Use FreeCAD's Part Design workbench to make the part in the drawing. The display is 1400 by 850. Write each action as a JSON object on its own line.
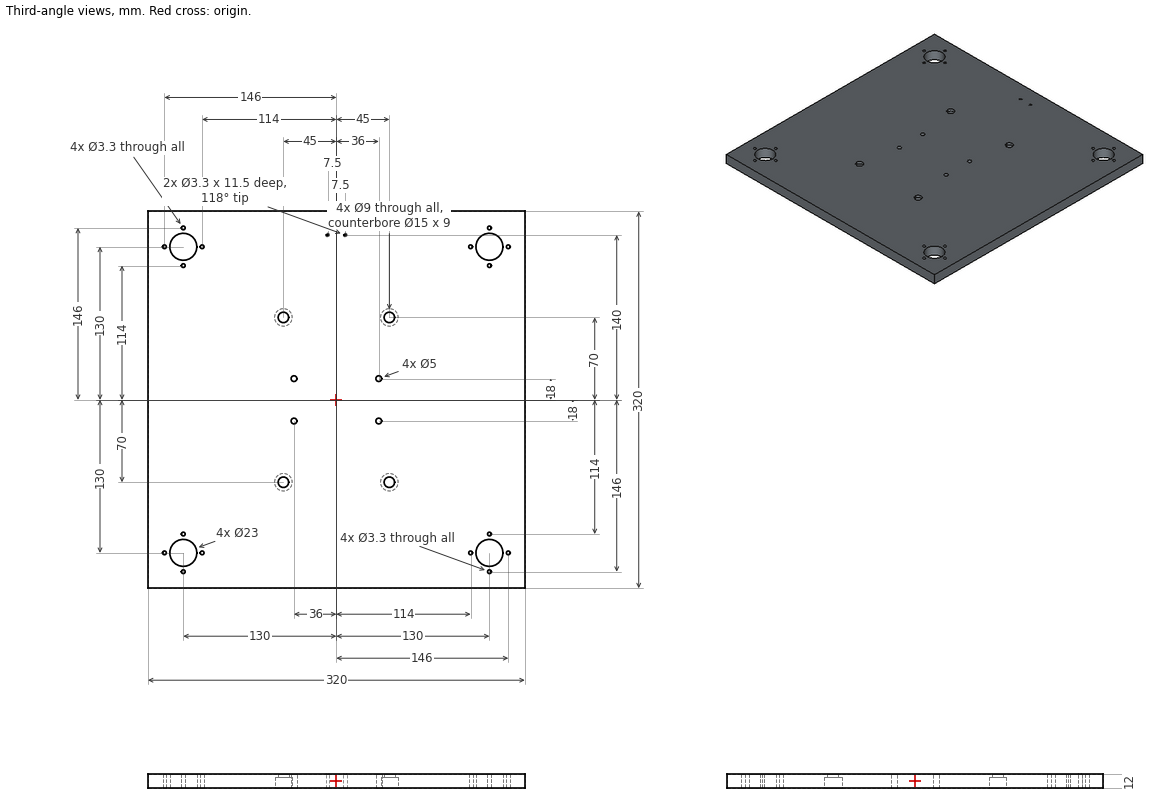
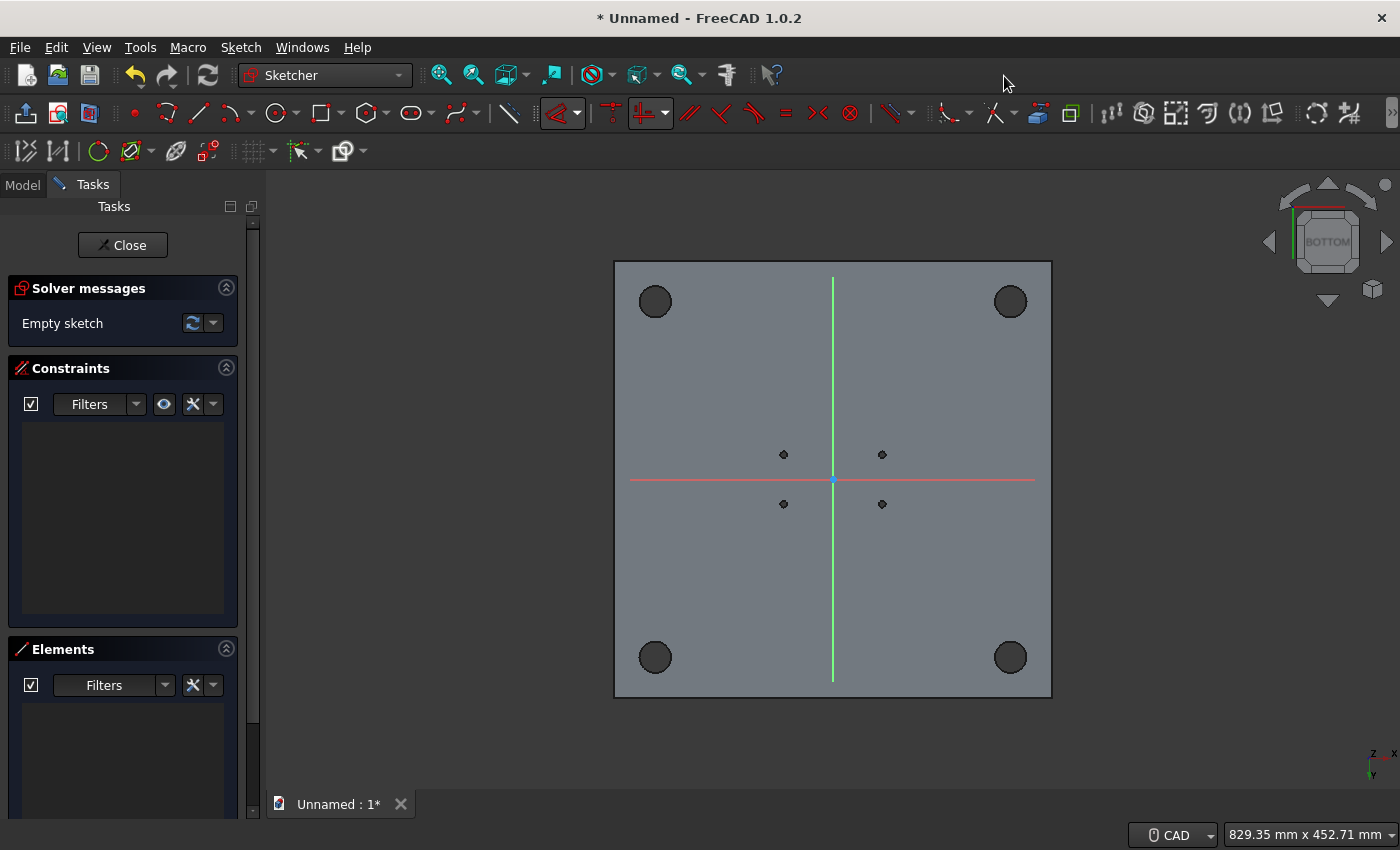
{"action": "scroll", "coordinate": [916, 480], "scroll_direction": "up", "scroll_amount": 3}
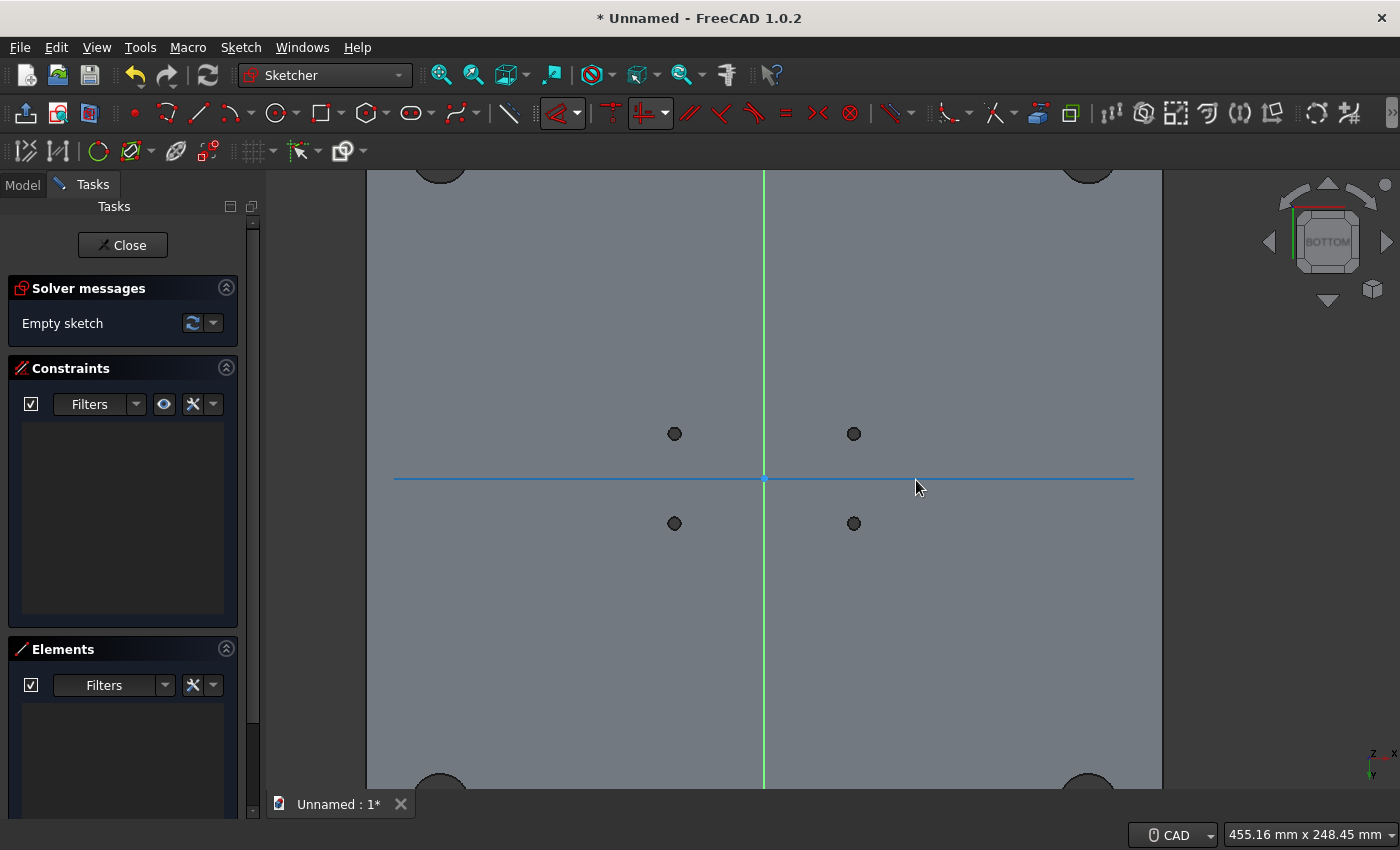
{"action": "left_click", "coordinate": [276, 114]}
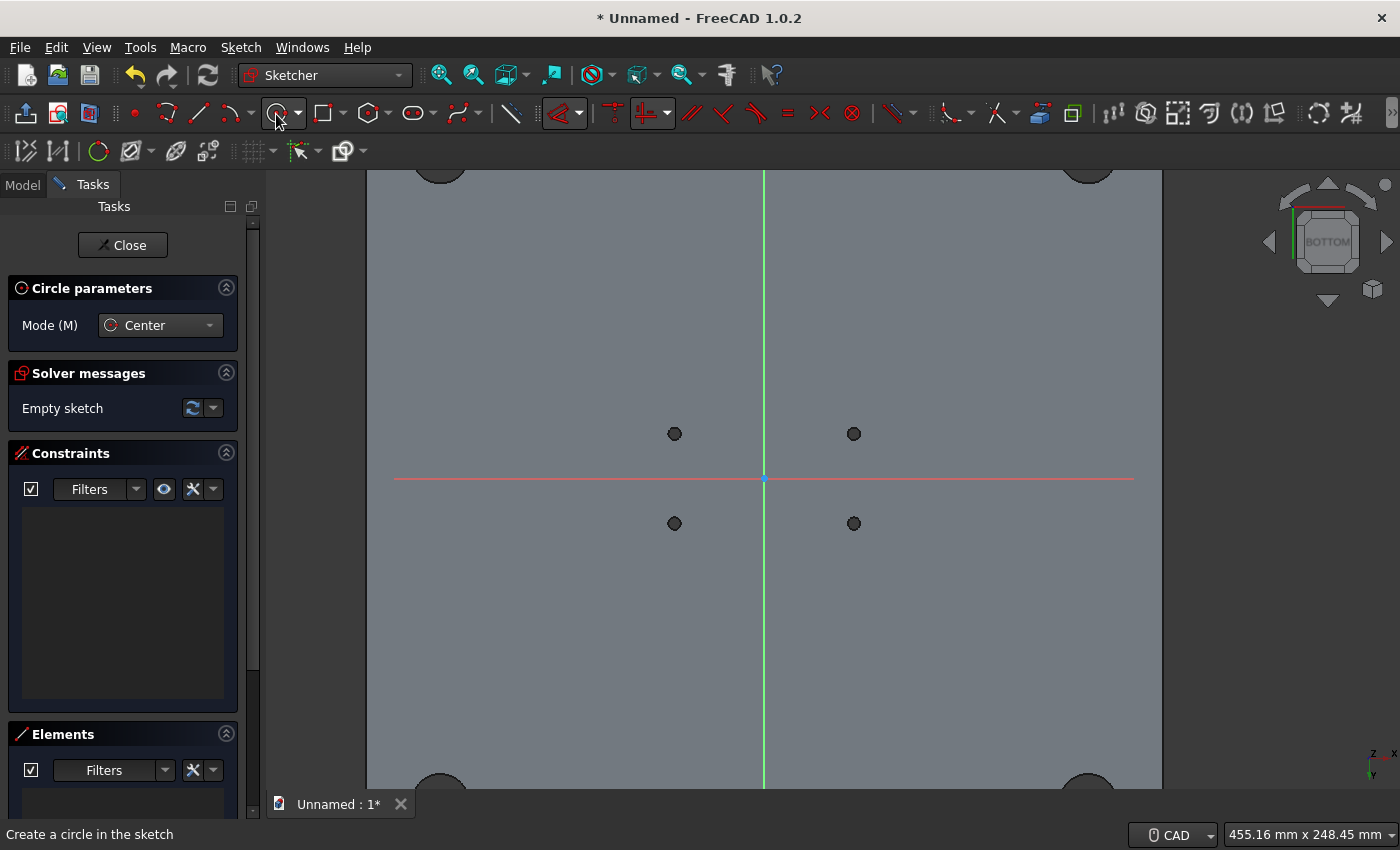
{"action": "scroll", "coordinate": [876, 653], "scroll_direction": "up", "scroll_amount": 4}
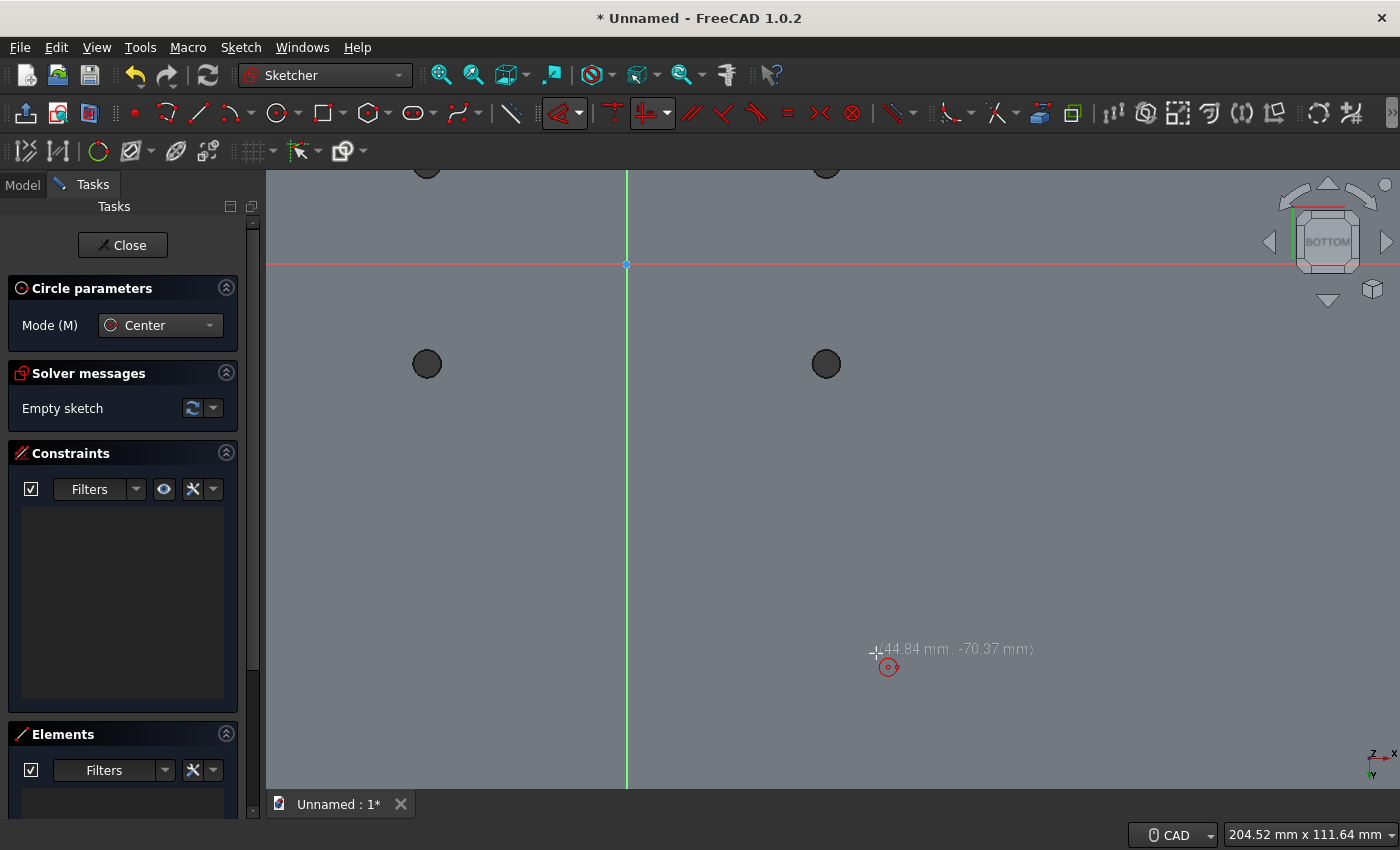
{"action": "left_click", "coordinate": [876, 652]}
{"action": "mouse_move", "coordinate": [894, 635]}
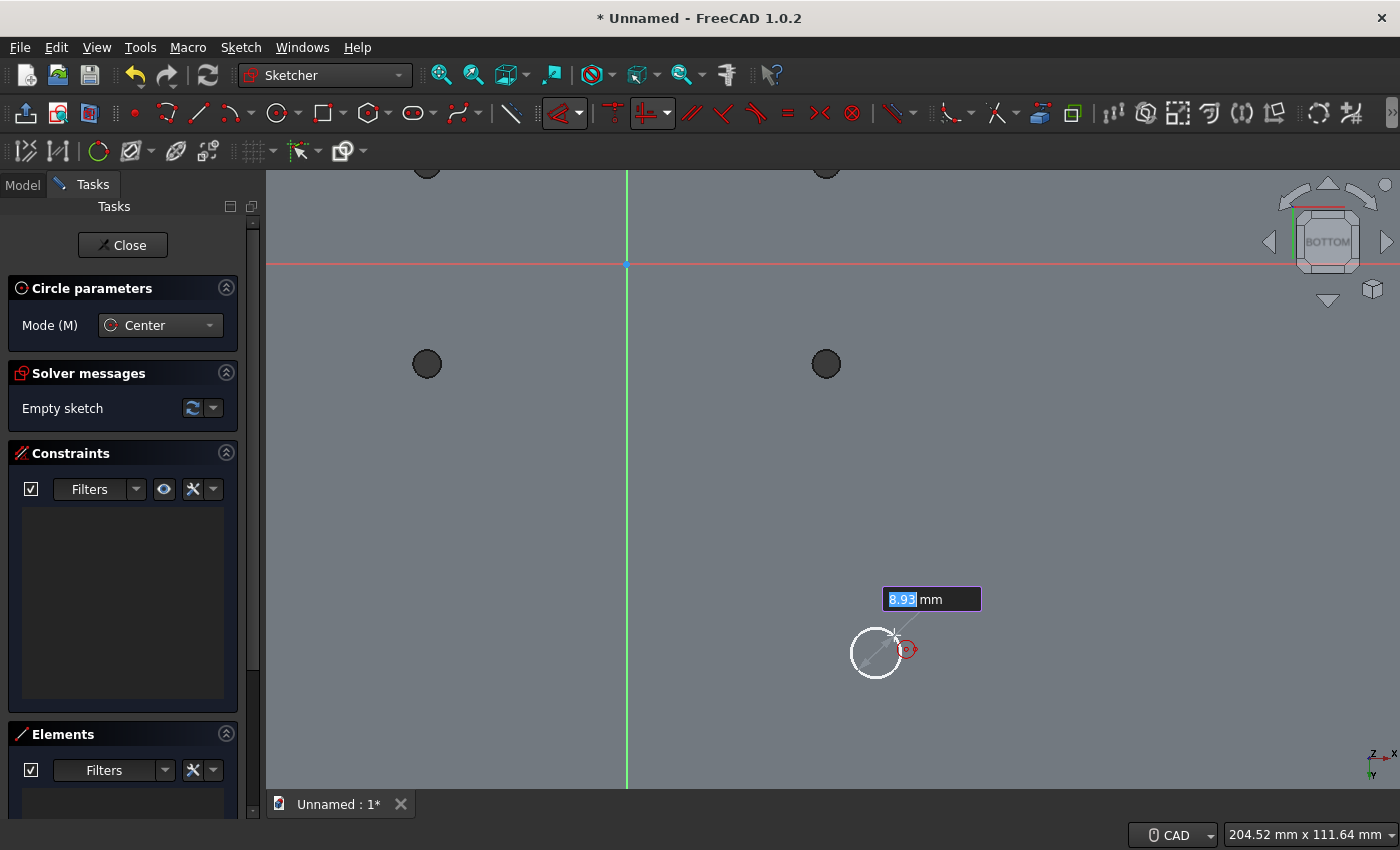
{"action": "type", "text": "9"}
{"action": "key", "text": "Return"}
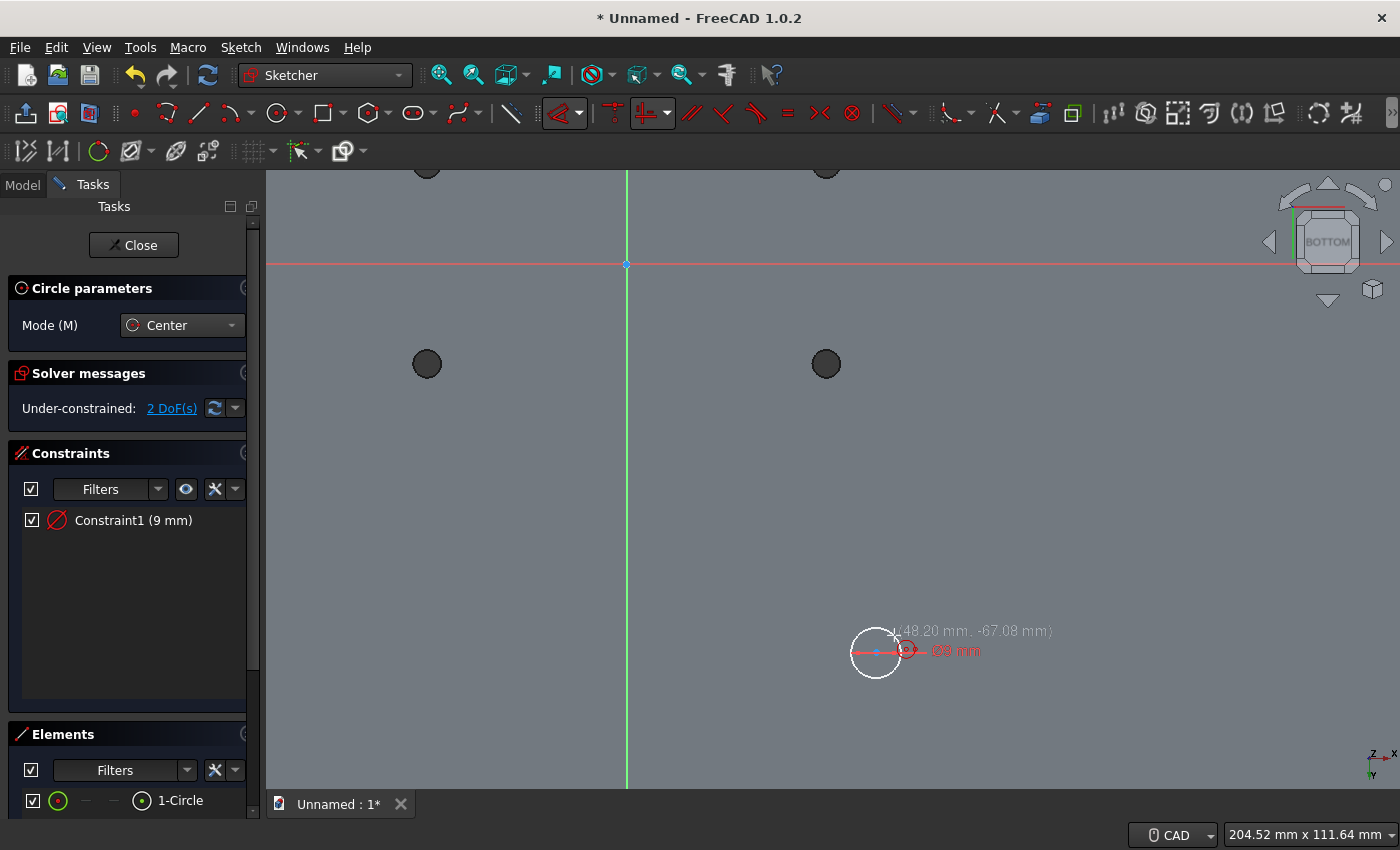
{"action": "left_click", "coordinate": [377, 652]}
{"action": "mouse_move", "coordinate": [395, 635]}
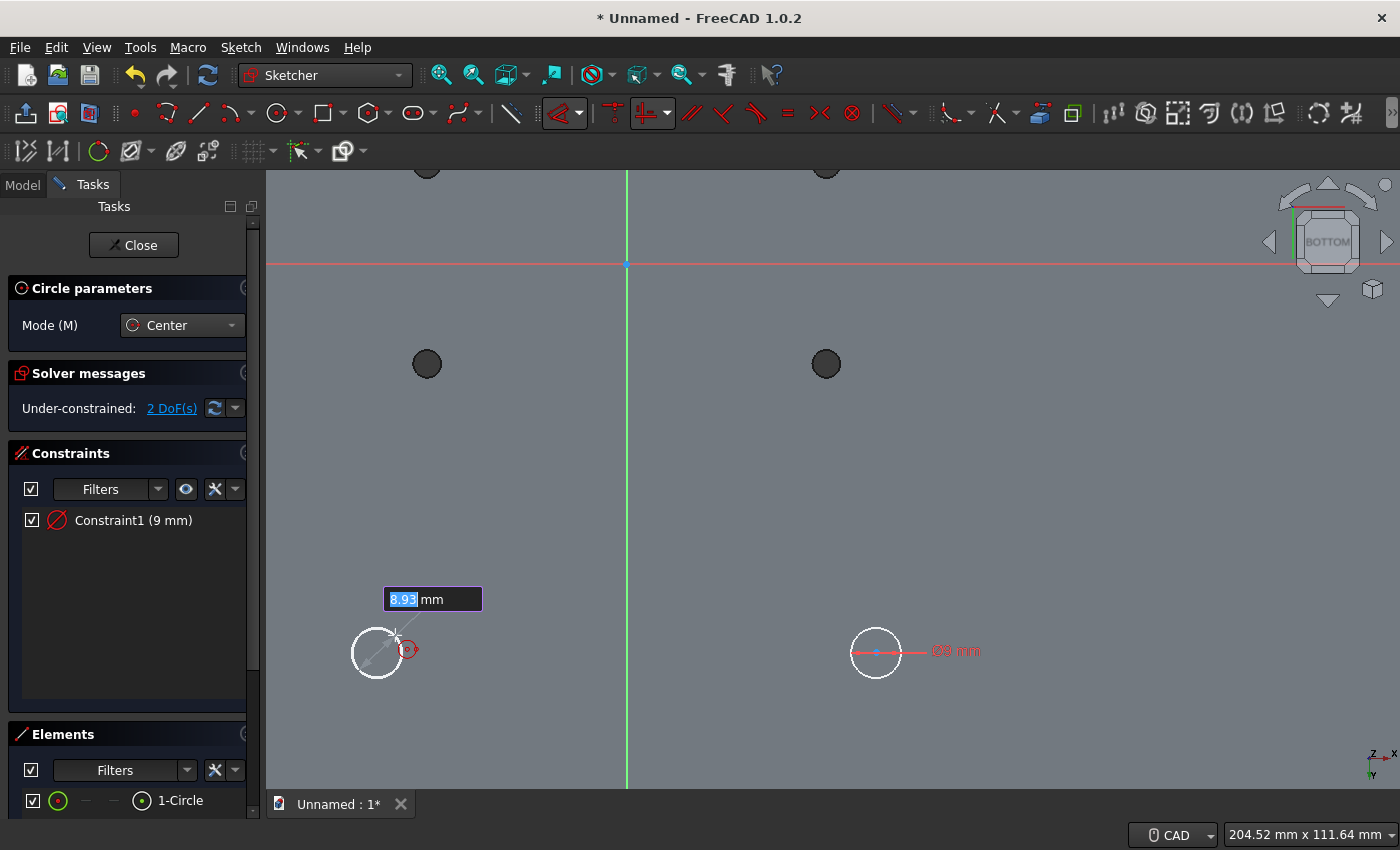
{"action": "type", "text": "9"}
{"action": "key", "text": "Return"}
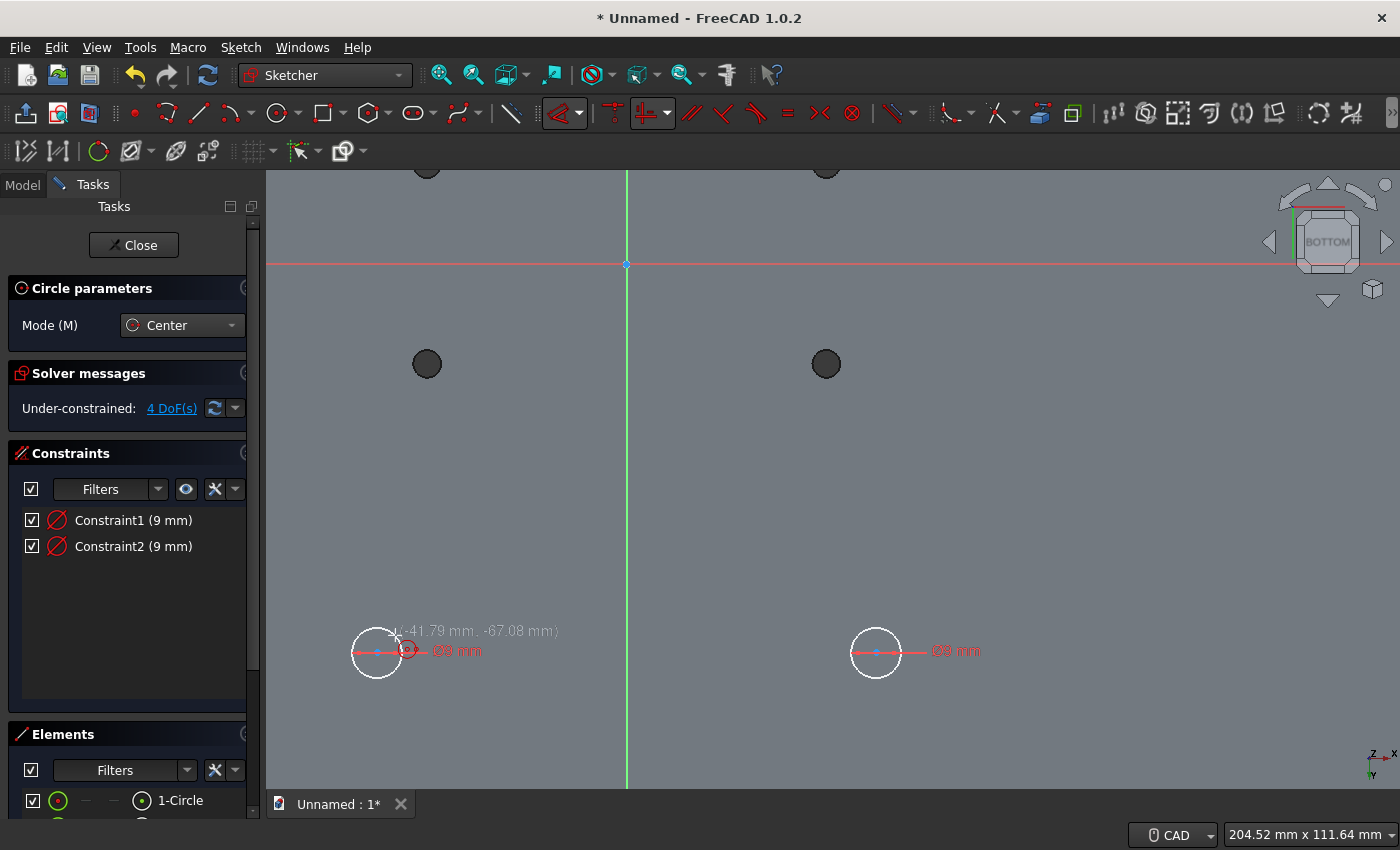
{"action": "scroll", "coordinate": [877, 655], "scroll_direction": "down", "scroll_amount": 4}